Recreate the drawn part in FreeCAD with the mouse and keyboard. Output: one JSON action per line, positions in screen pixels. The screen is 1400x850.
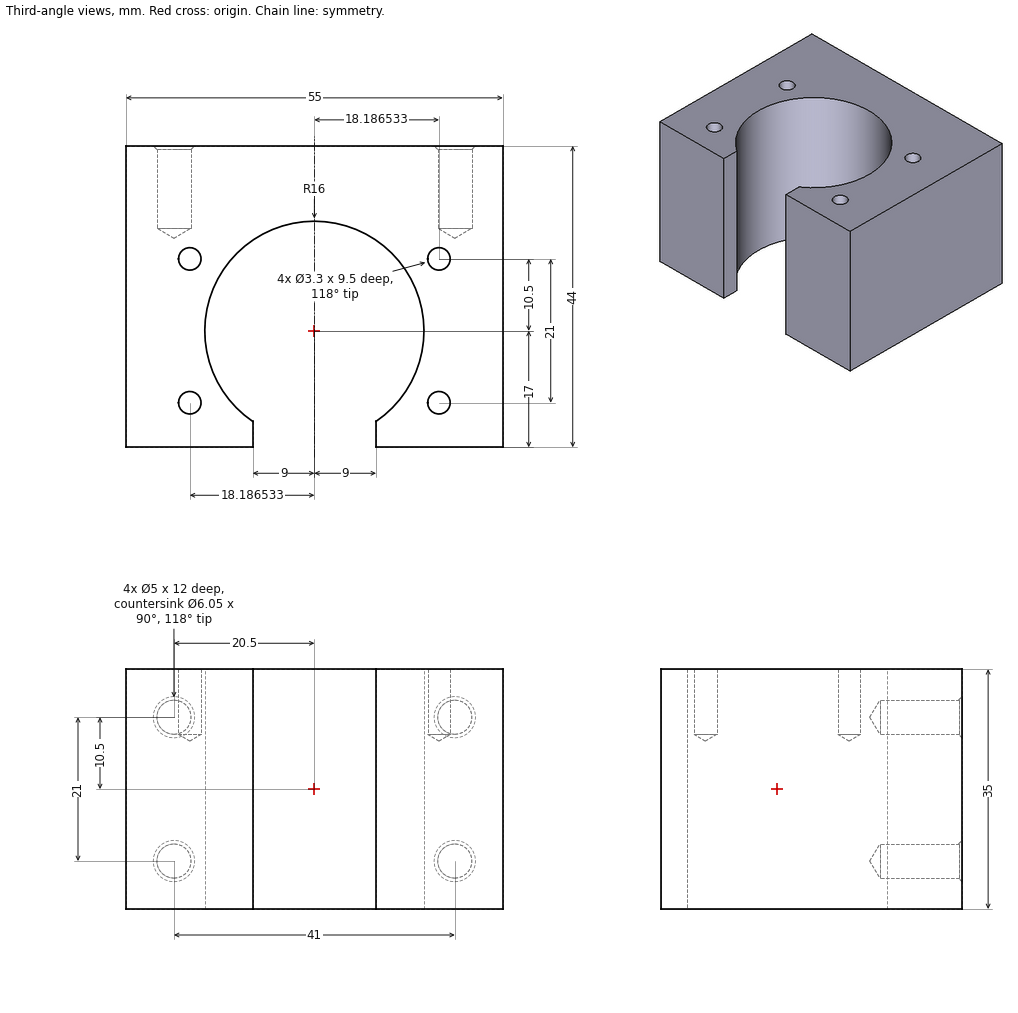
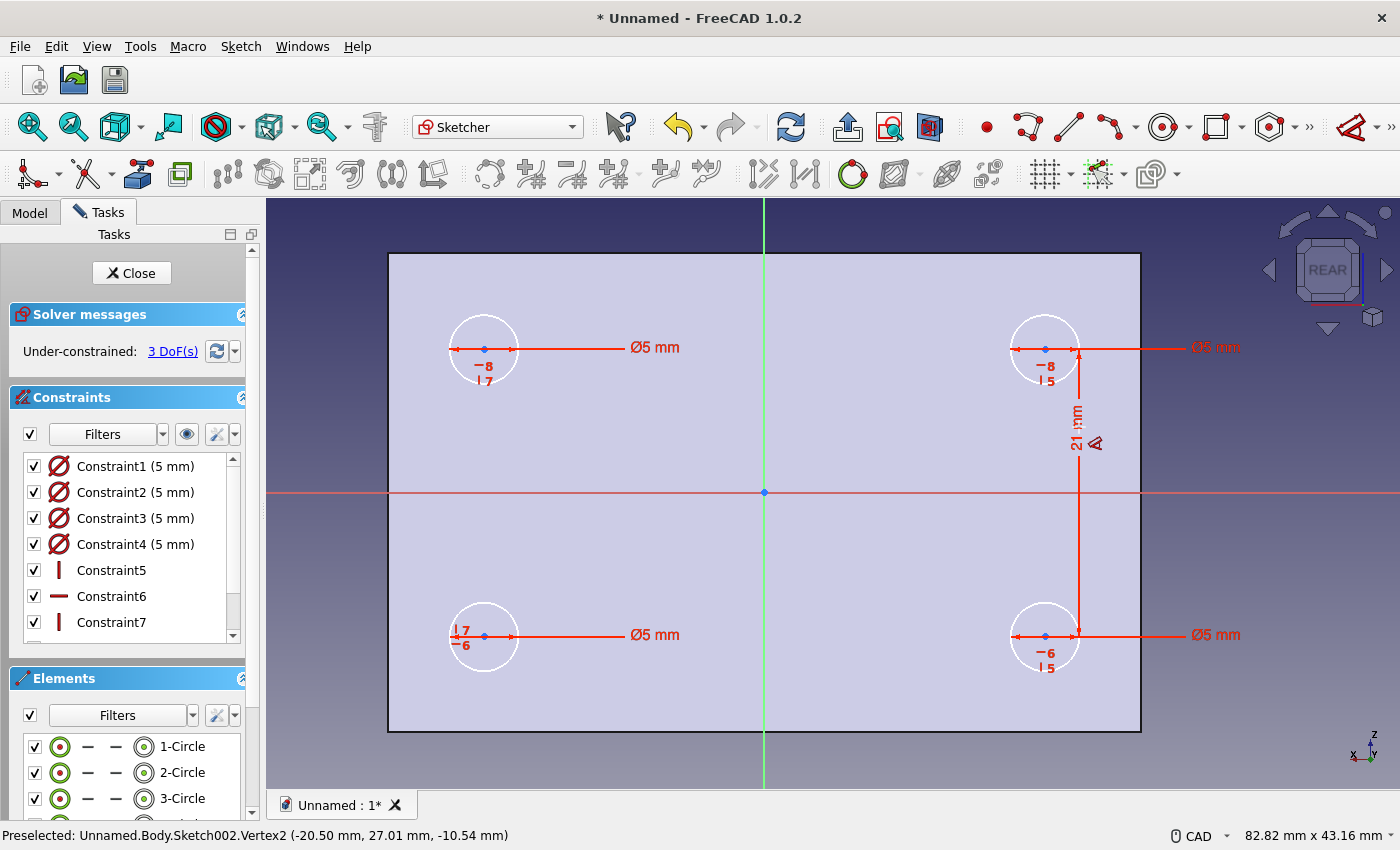
{"action": "left_click", "coordinate": [1045, 637]}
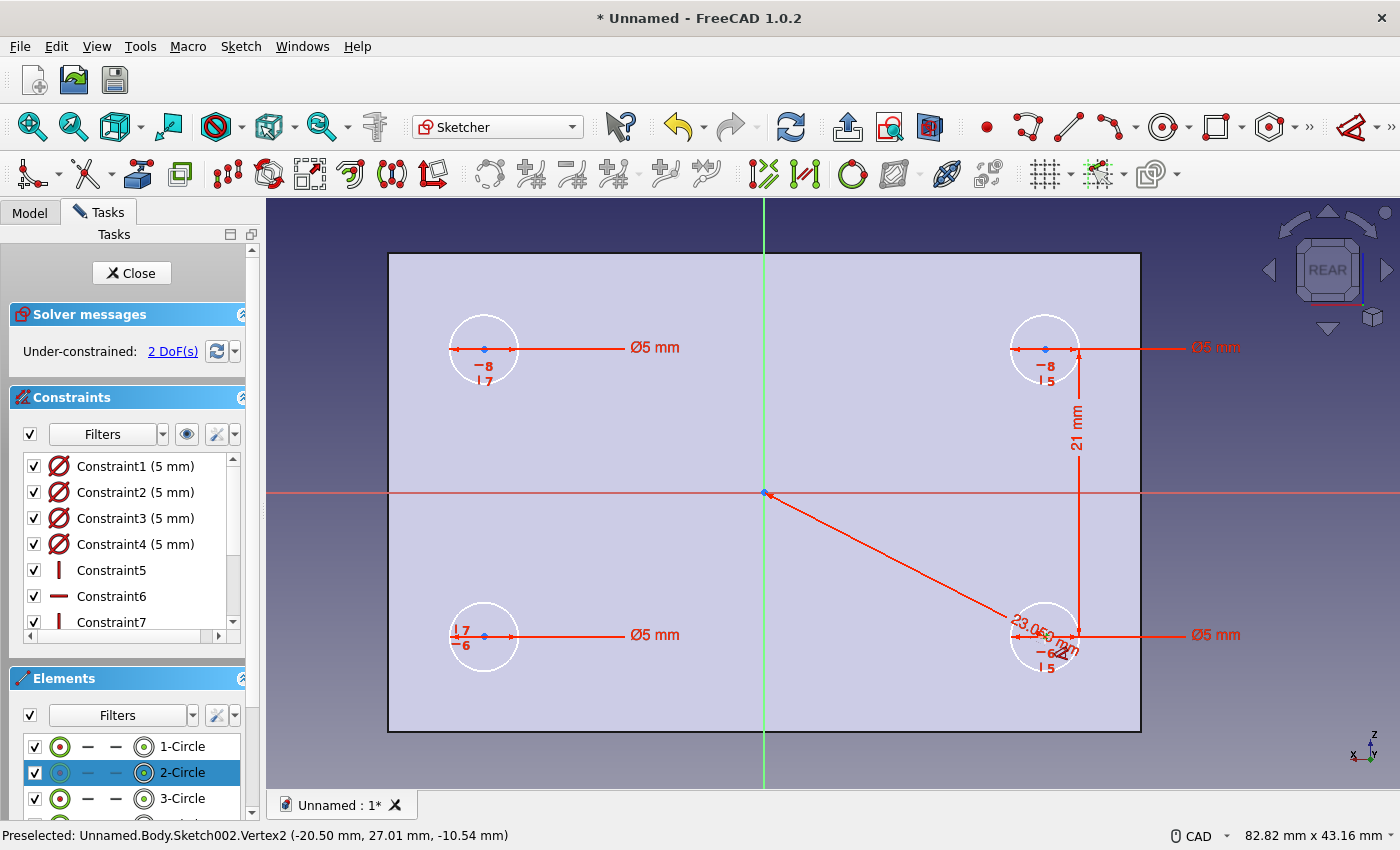
{"action": "left_click", "coordinate": [484, 637]}
{"action": "left_click", "coordinate": [635, 671]}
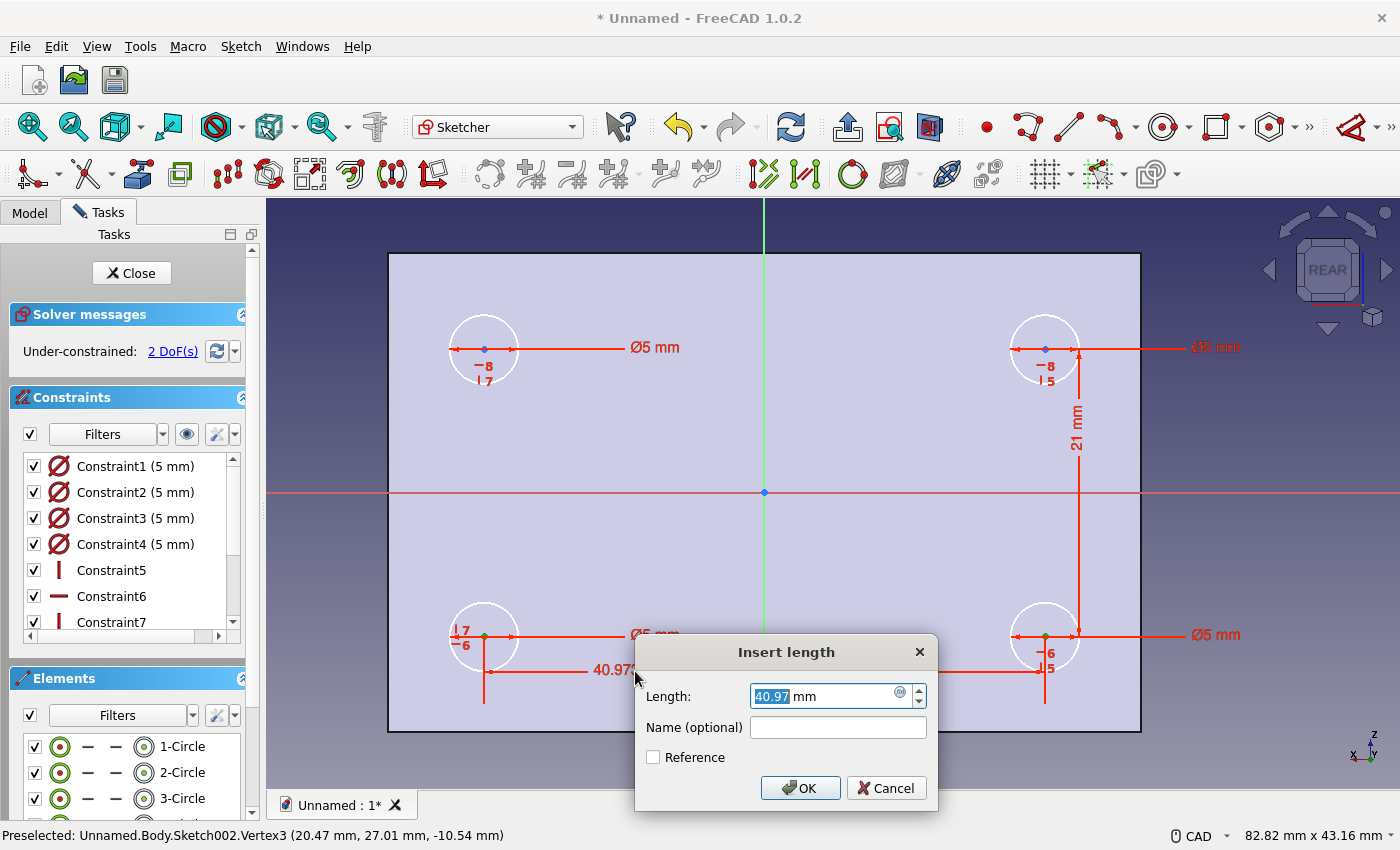
{"action": "type", "text": "41"}
{"action": "key", "text": "Return"}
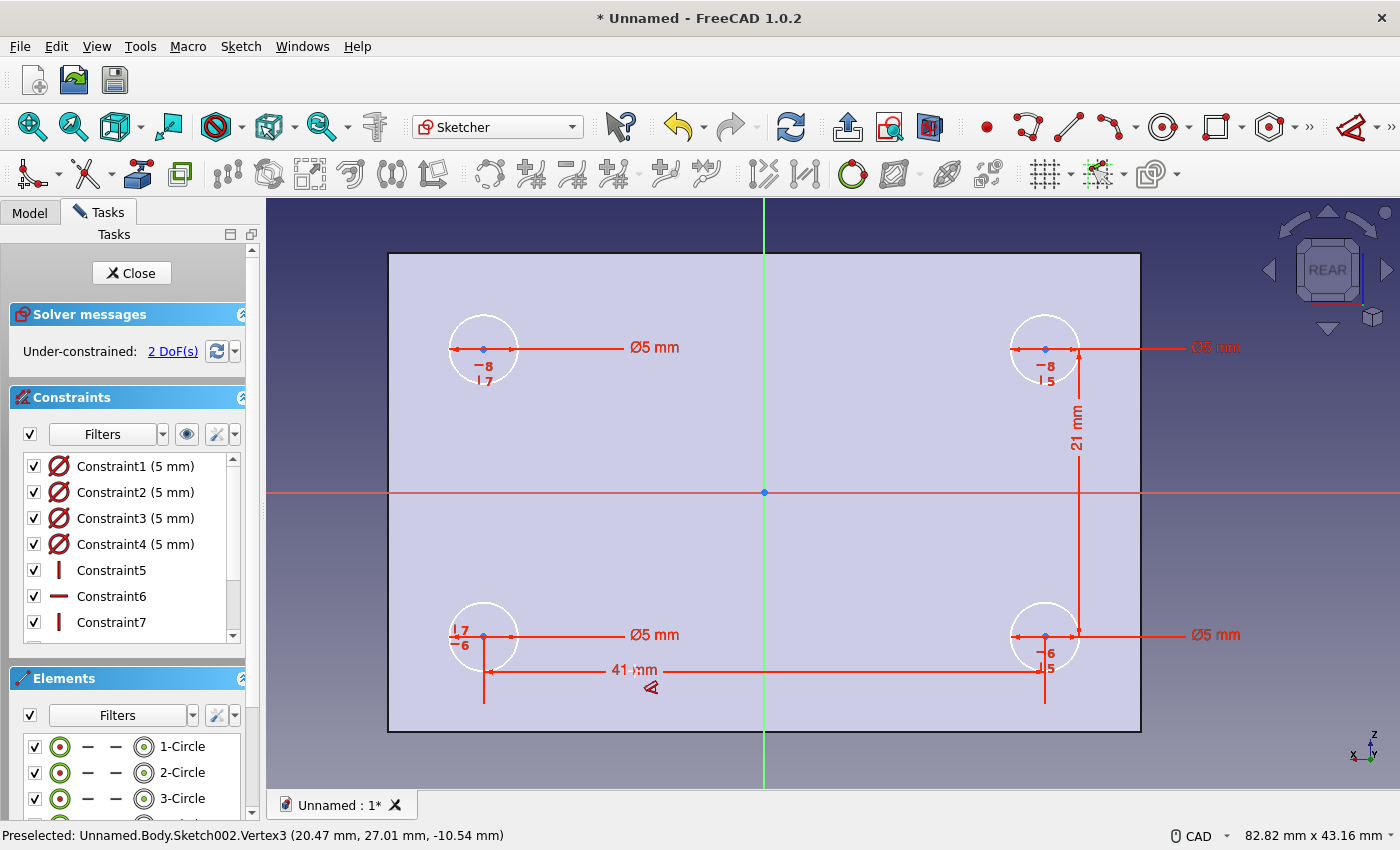
{"action": "left_click", "coordinate": [1045, 349]}
{"action": "left_click", "coordinate": [905, 315]}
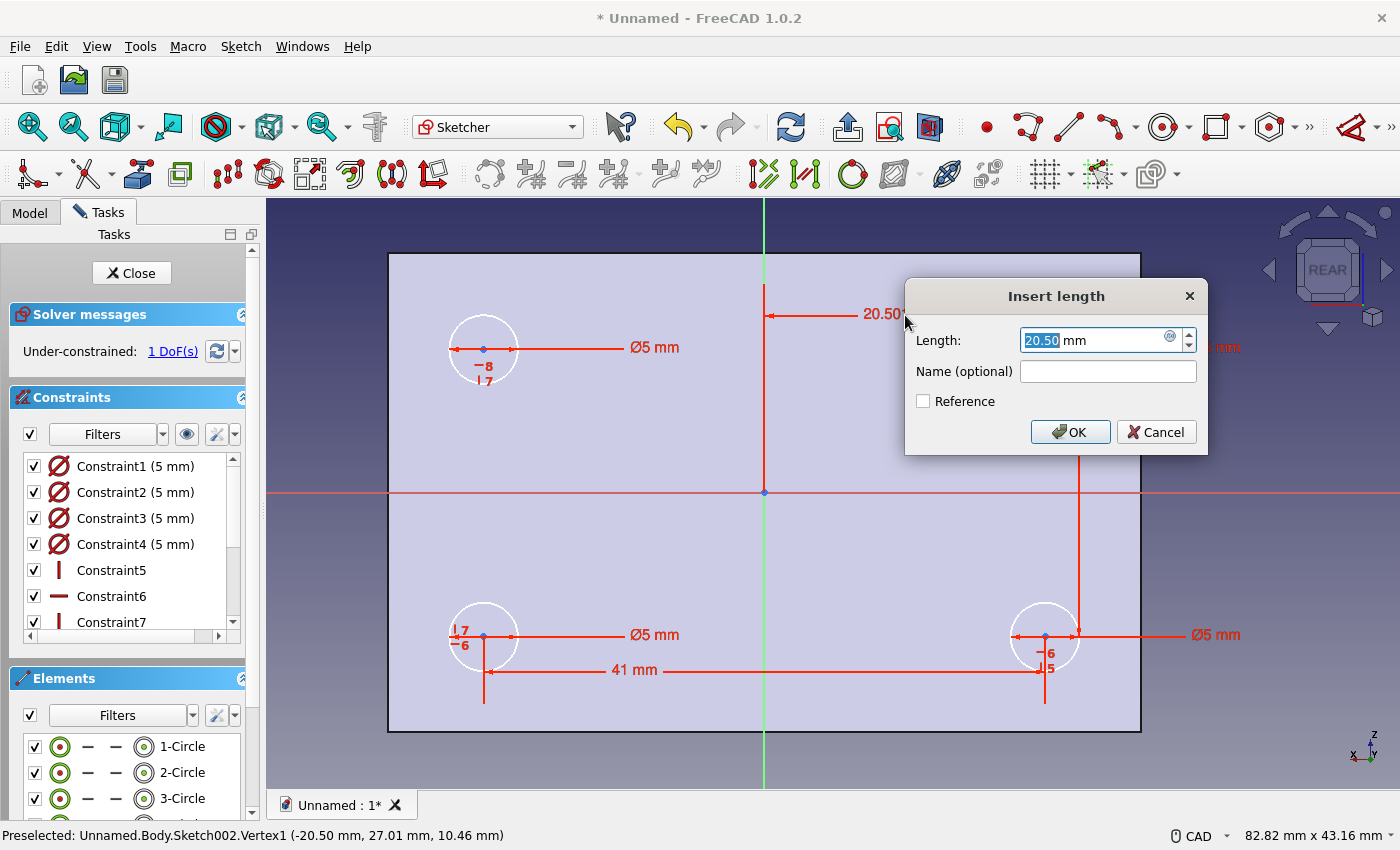
{"action": "type", "text": "20.5"}
{"action": "key", "text": "Return"}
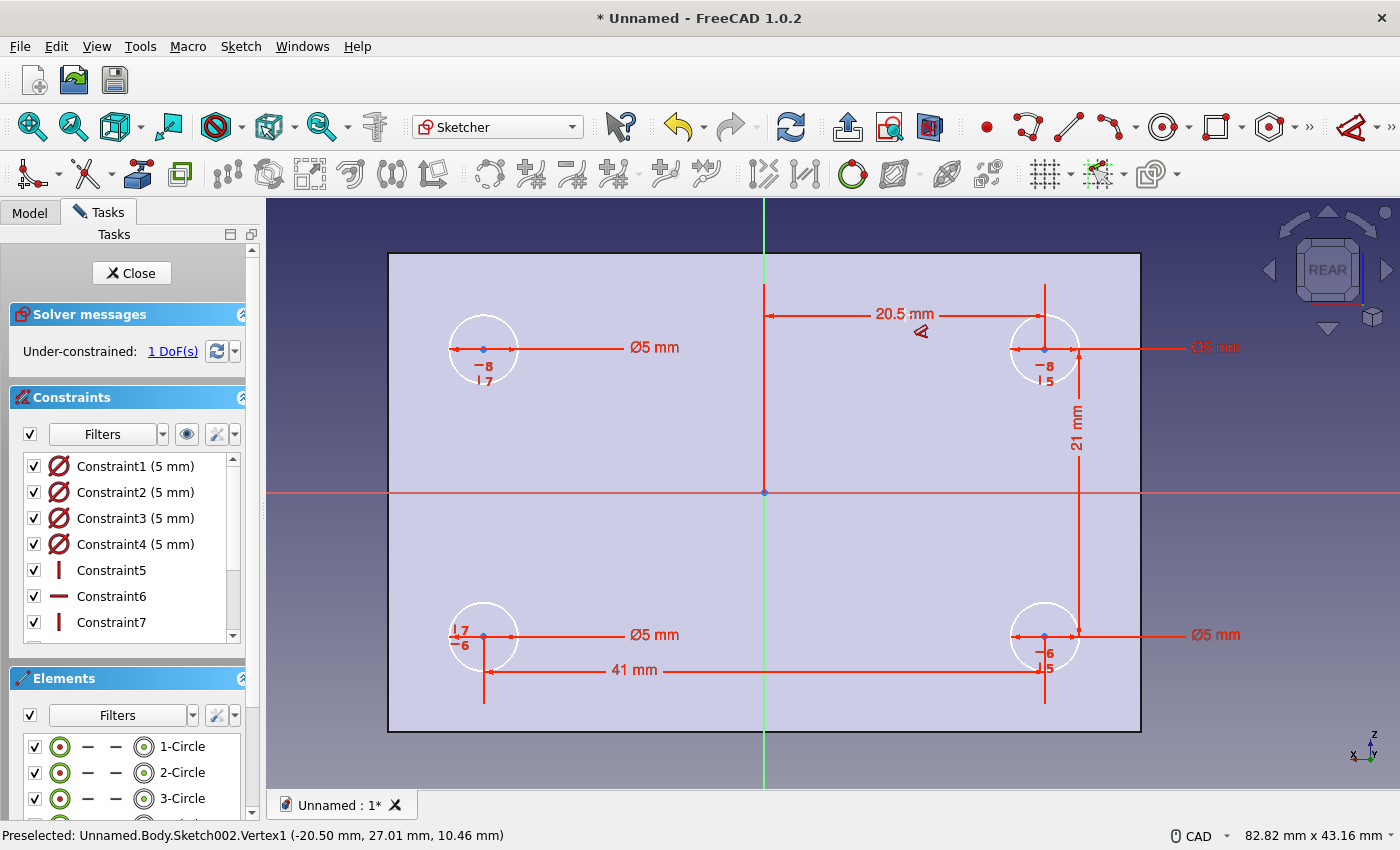
{"action": "left_click", "coordinate": [1045, 349]}
{"action": "left_click", "coordinate": [1079, 388]}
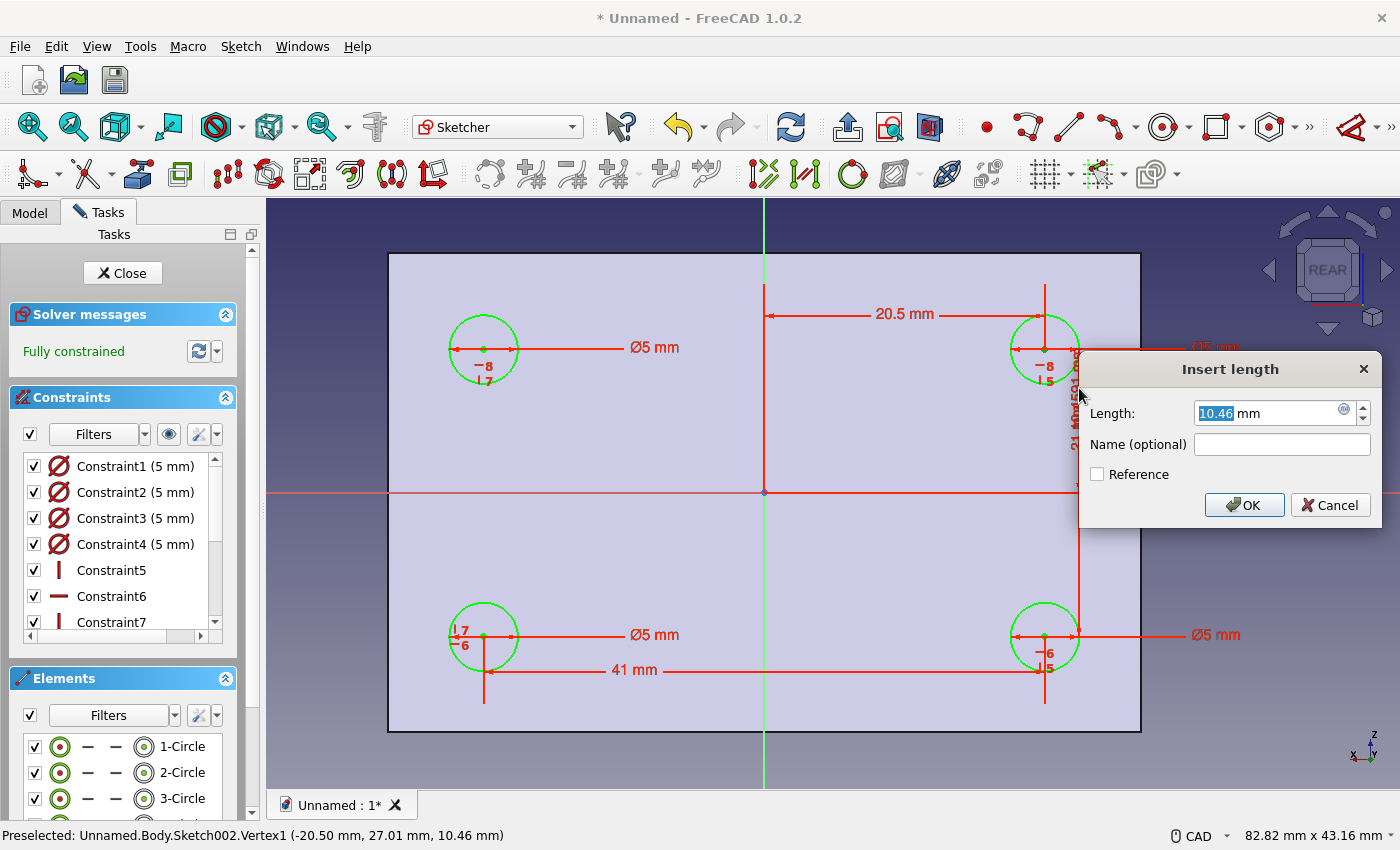
{"action": "type", "text": "10.5"}
{"action": "key", "text": "Return"}
{"action": "key", "text": "Escape"}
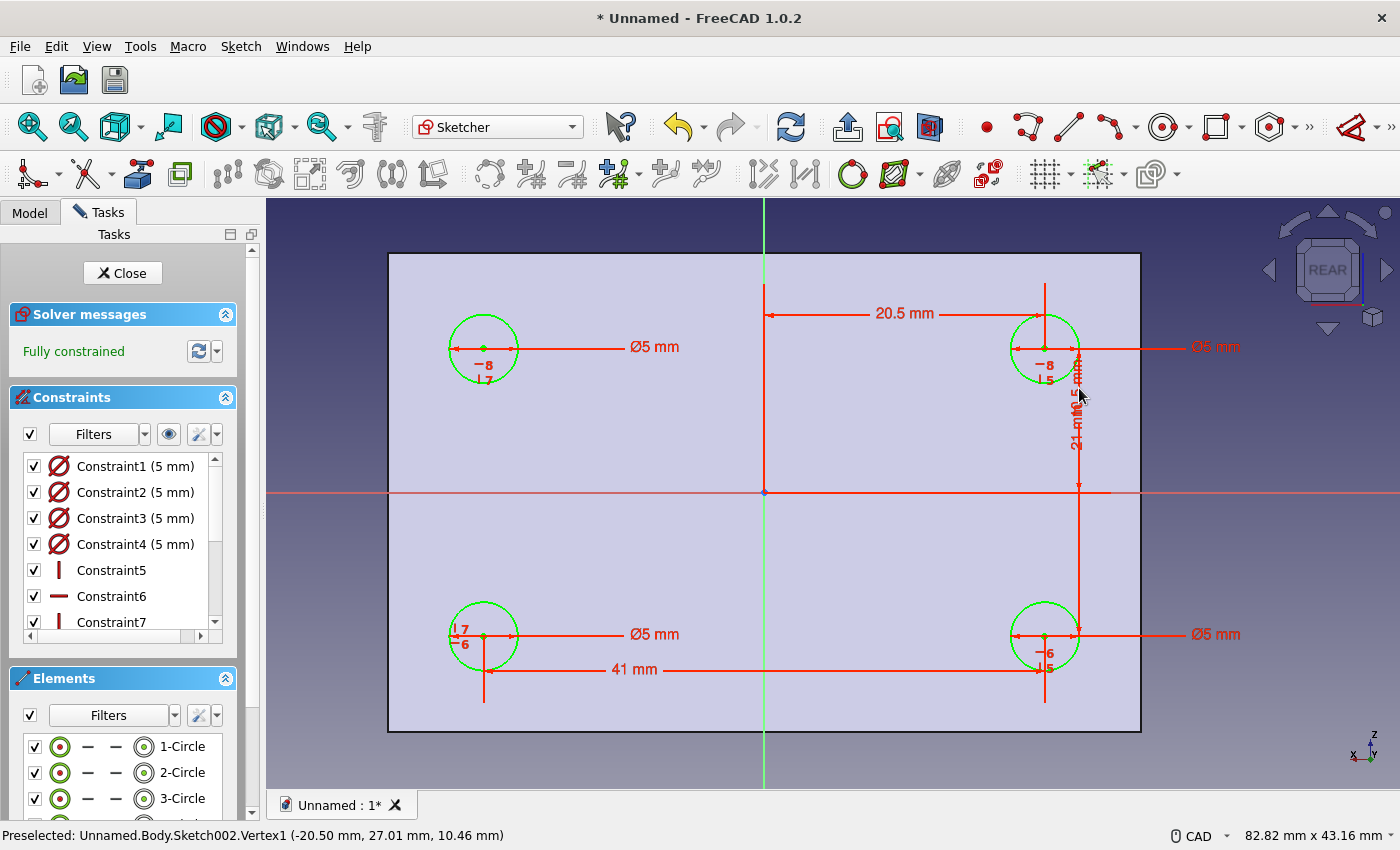
{"action": "left_click", "coordinate": [123, 273]}